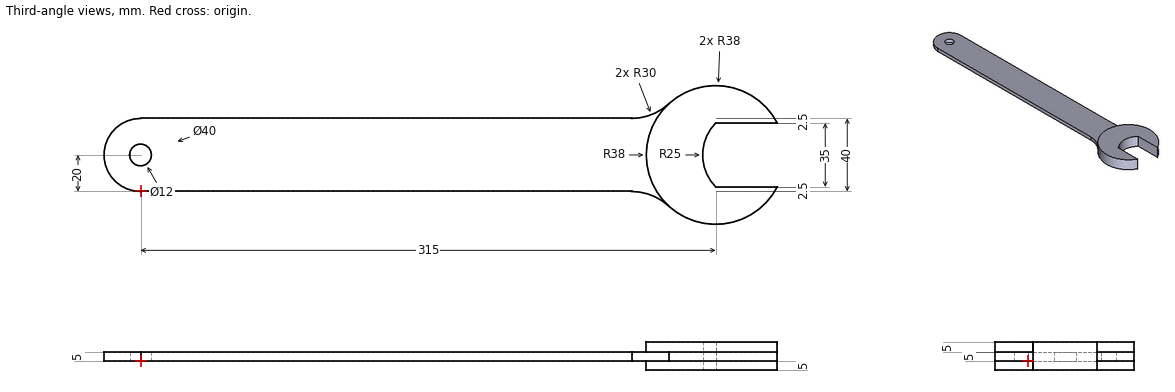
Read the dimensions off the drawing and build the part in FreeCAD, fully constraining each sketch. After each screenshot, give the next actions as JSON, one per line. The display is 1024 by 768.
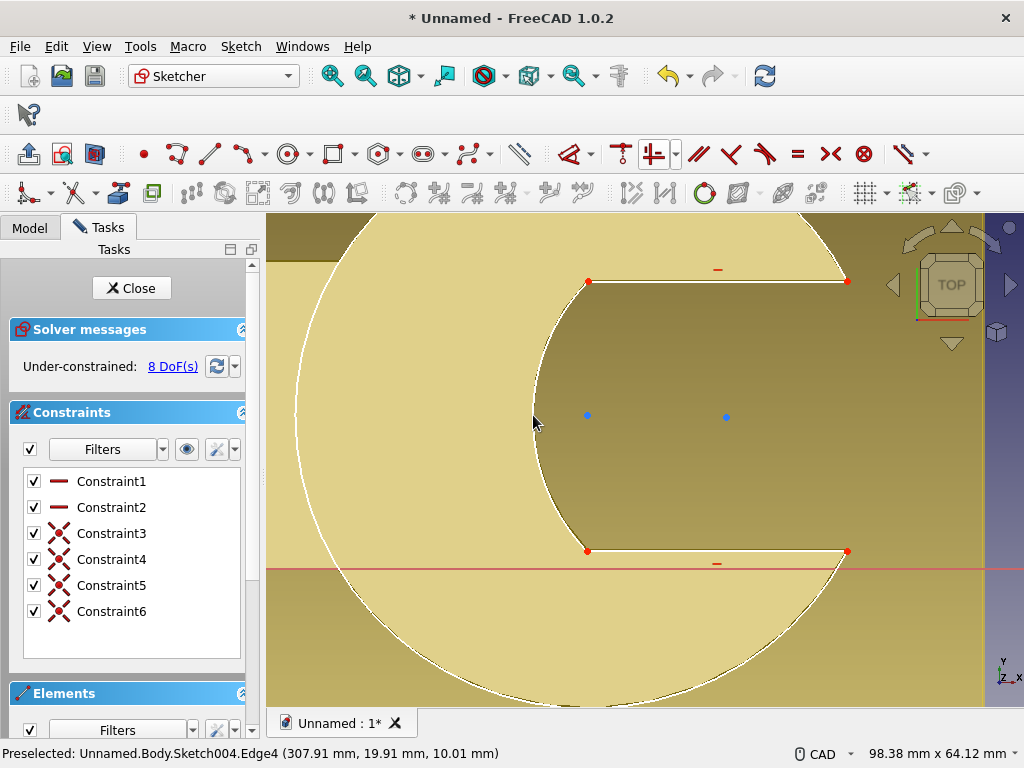
{"action": "left_click", "coordinate": [568, 154]}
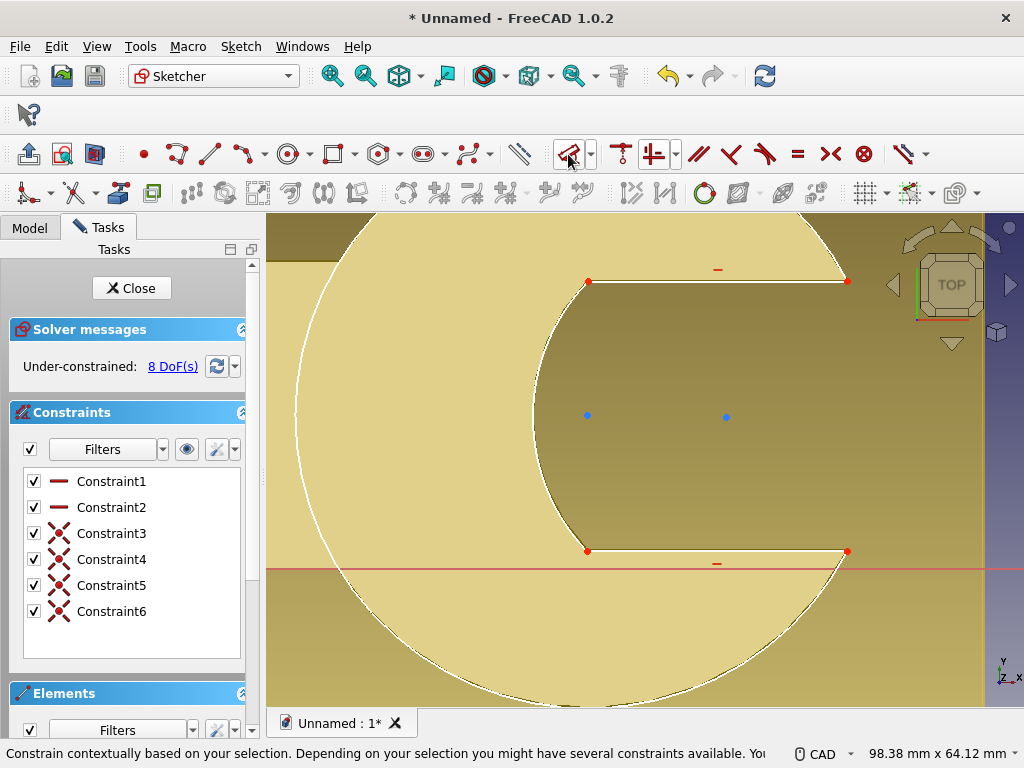
{"action": "left_click", "coordinate": [446, 671]}
{"action": "left_click", "coordinate": [314, 589]}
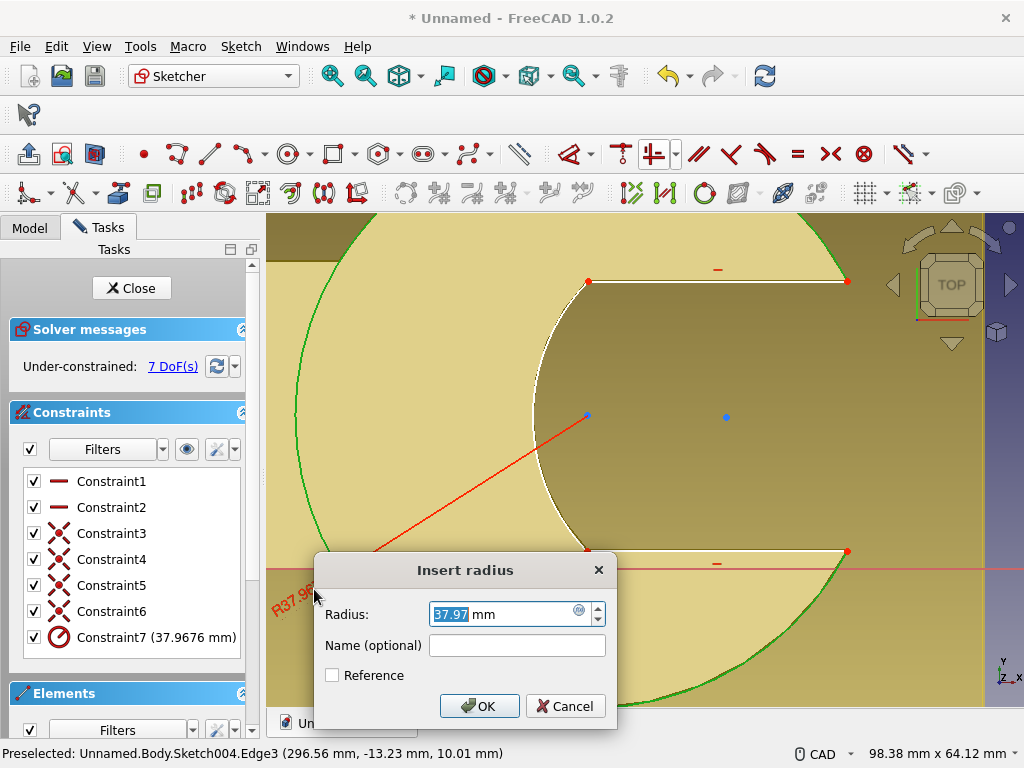
{"action": "type", "text": "38"}
{"action": "key", "text": "Return"}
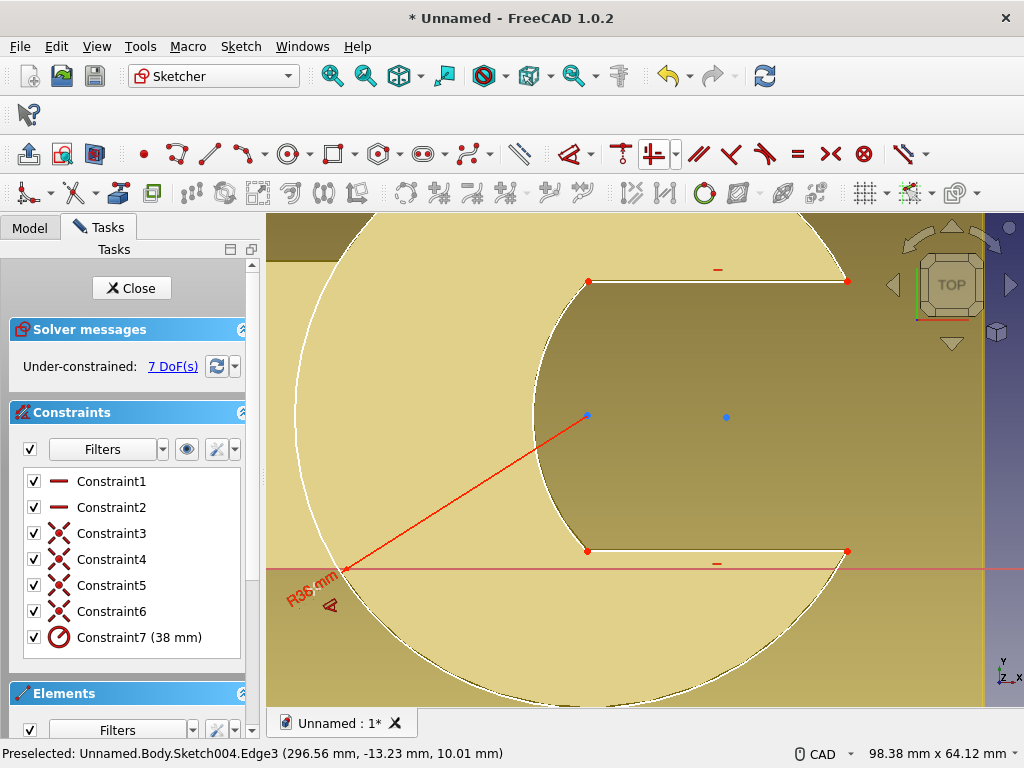
{"action": "left_click", "coordinate": [542, 358]}
{"action": "left_click", "coordinate": [512, 348]}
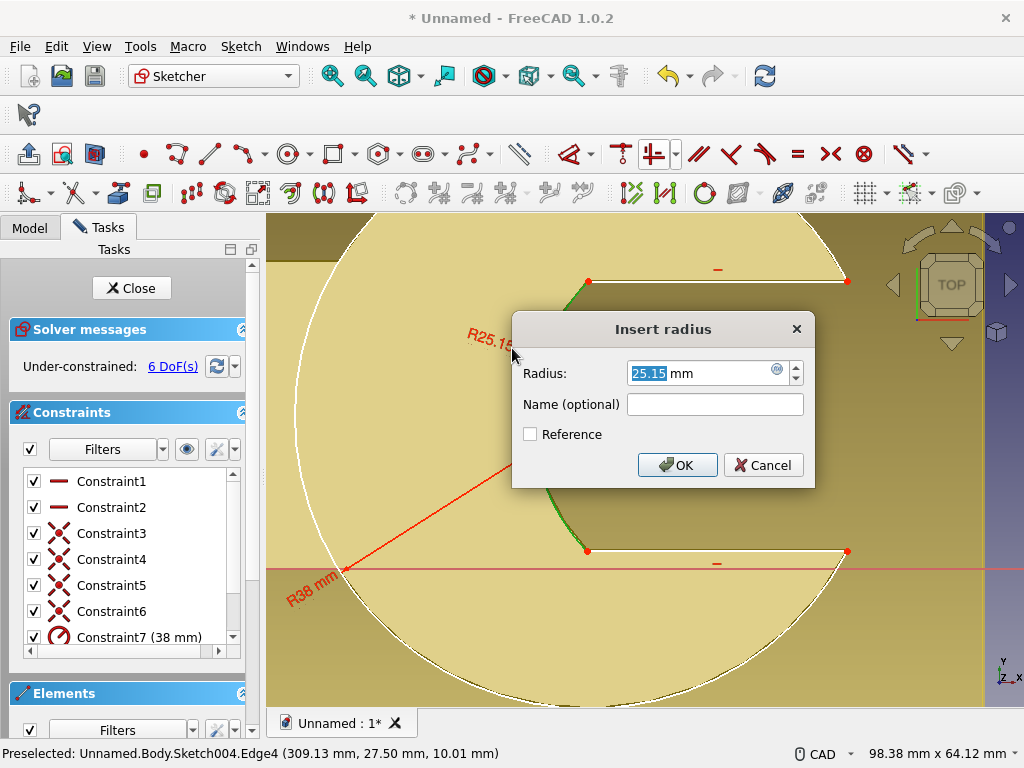
{"action": "type", "text": "25"}
{"action": "key", "text": "Return"}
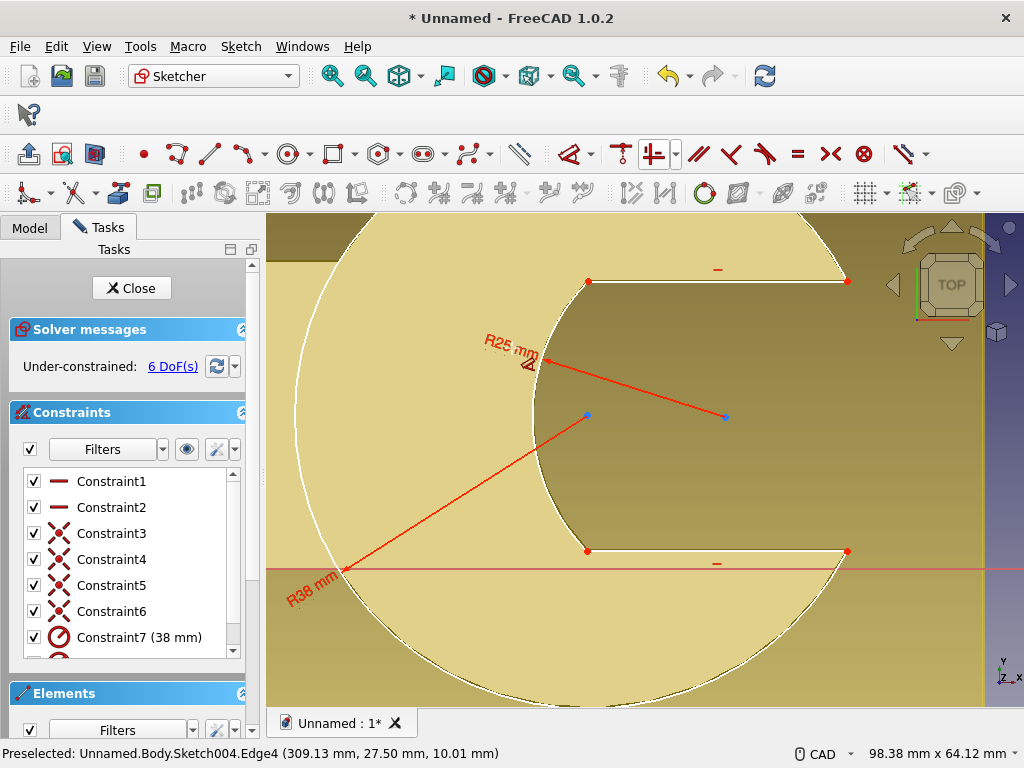
{"action": "left_click", "coordinate": [588, 416]}
{"action": "left_click", "coordinate": [622, 493]}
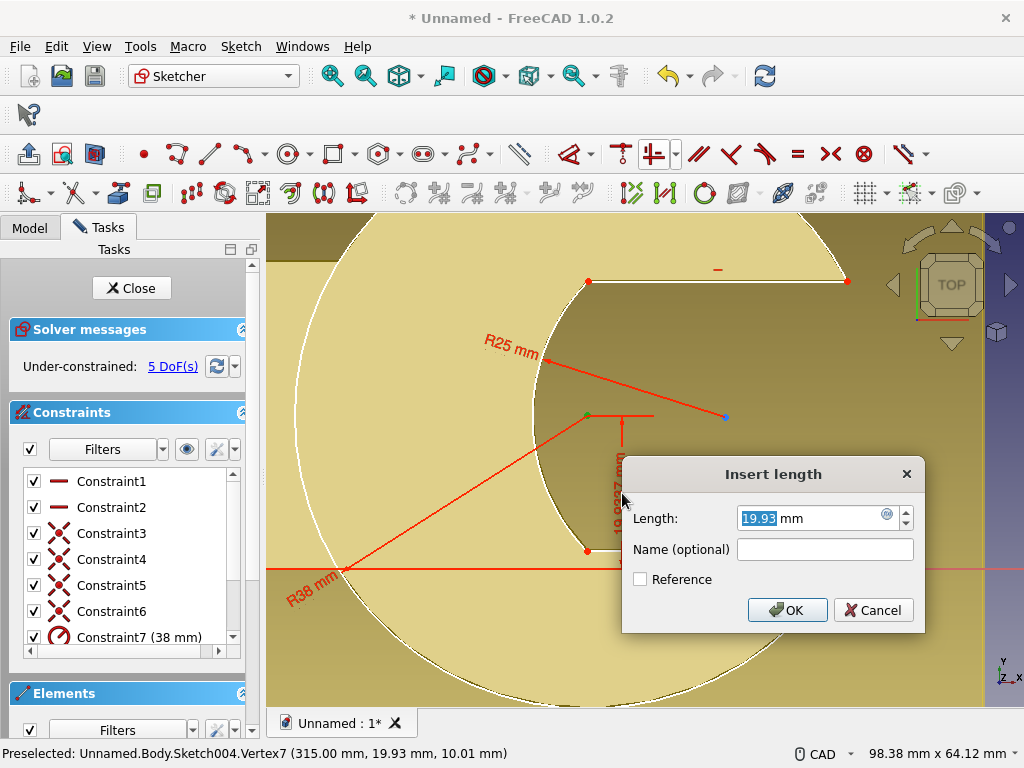
{"action": "type", "text": "20"}
{"action": "key", "text": "Return"}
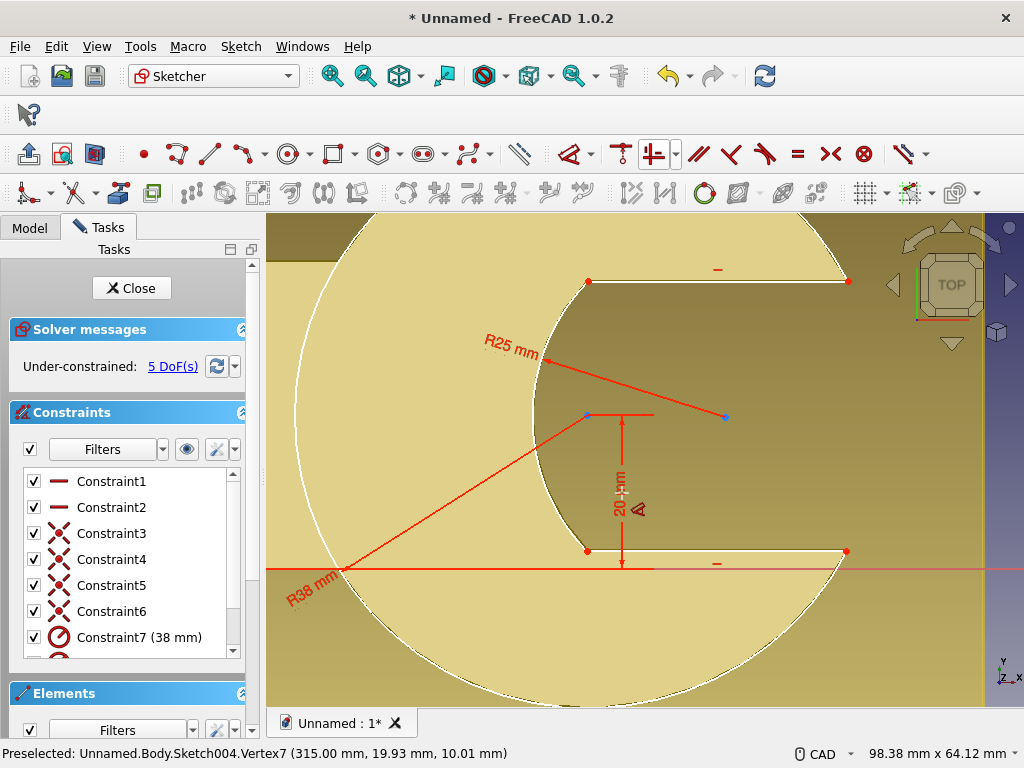
{"action": "left_click", "coordinate": [725, 417]}
{"action": "left_click", "coordinate": [759, 493]}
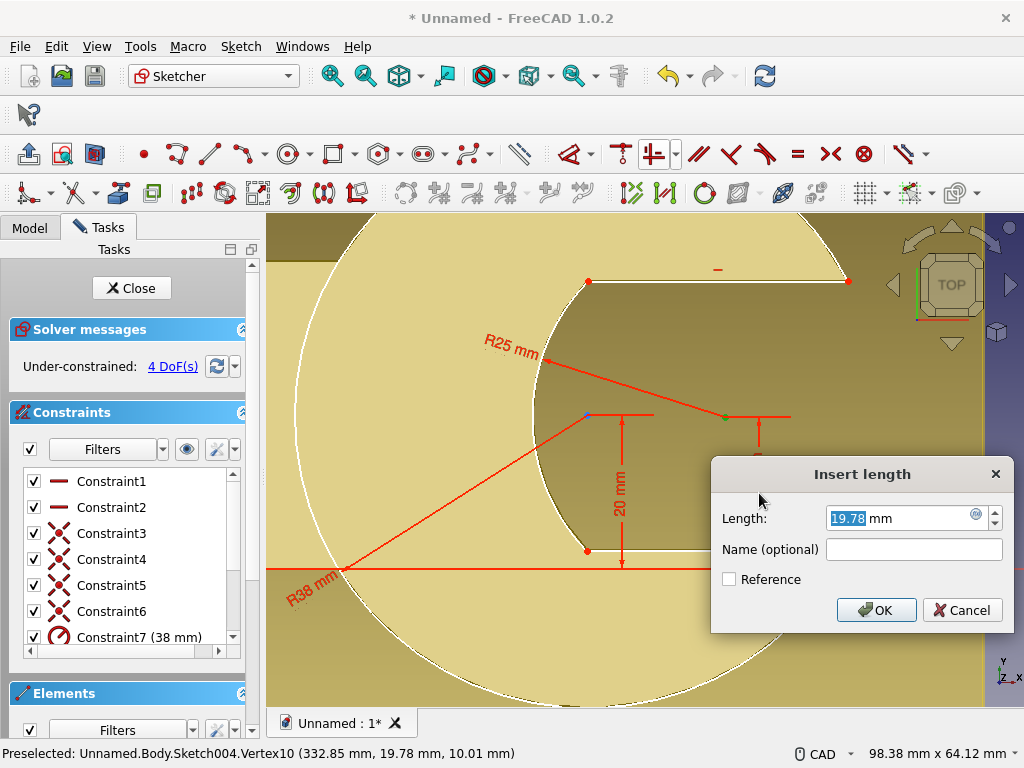
{"action": "type", "text": "20"}
{"action": "key", "text": "Return"}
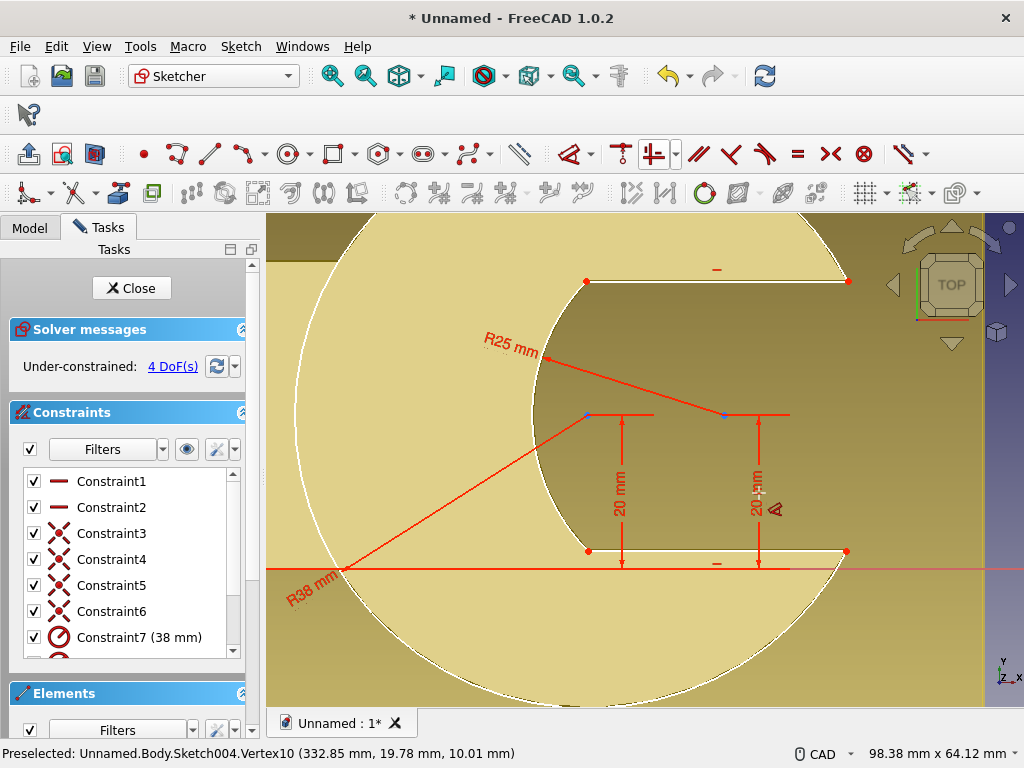
{"action": "left_click", "coordinate": [586, 282]}
{"action": "left_click", "coordinate": [440, 603]}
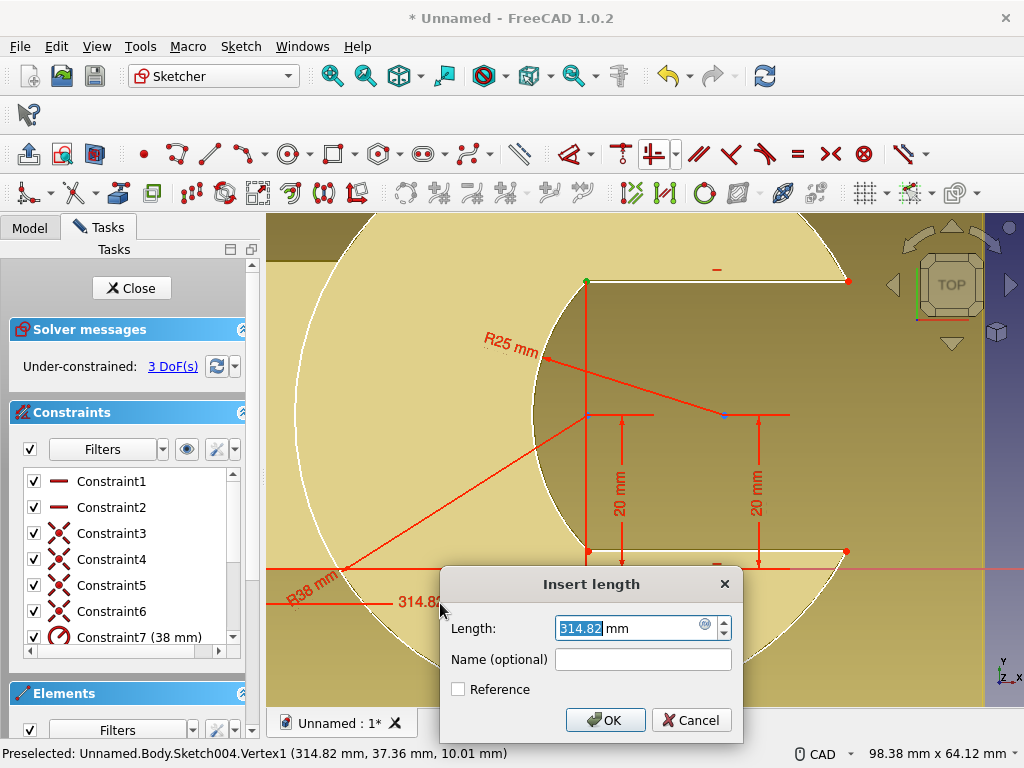
{"action": "type", "text": "315"}
{"action": "key", "text": "Return"}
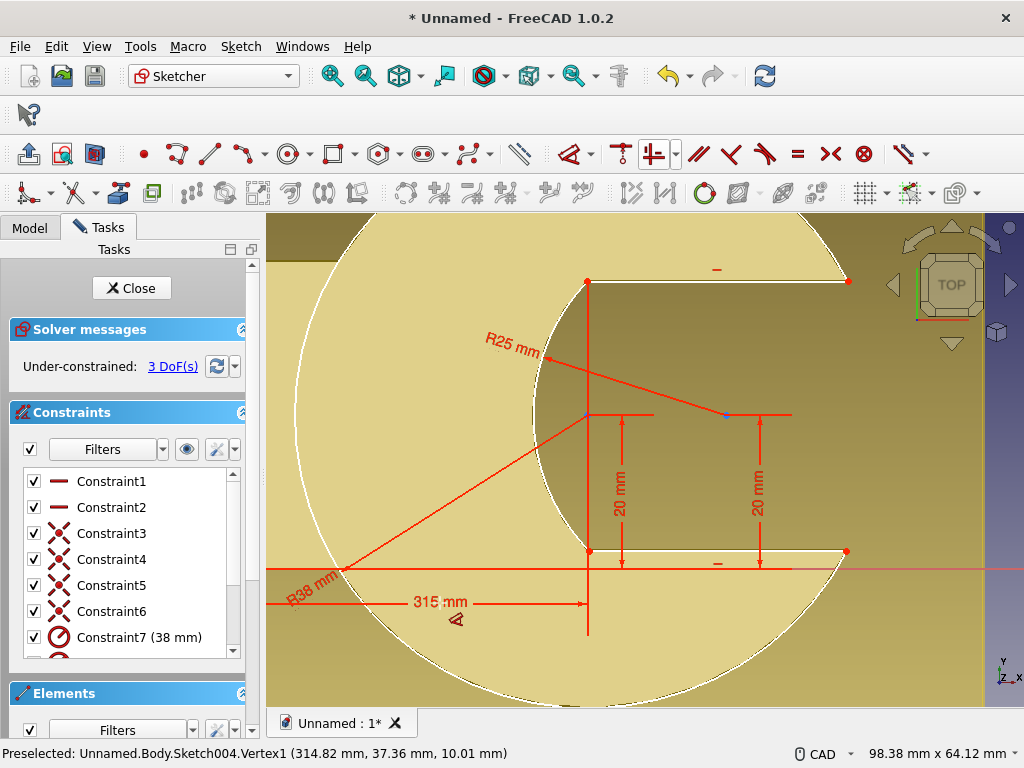
{"action": "scroll", "coordinate": [847, 551], "scroll_direction": "up", "scroll_amount": 4}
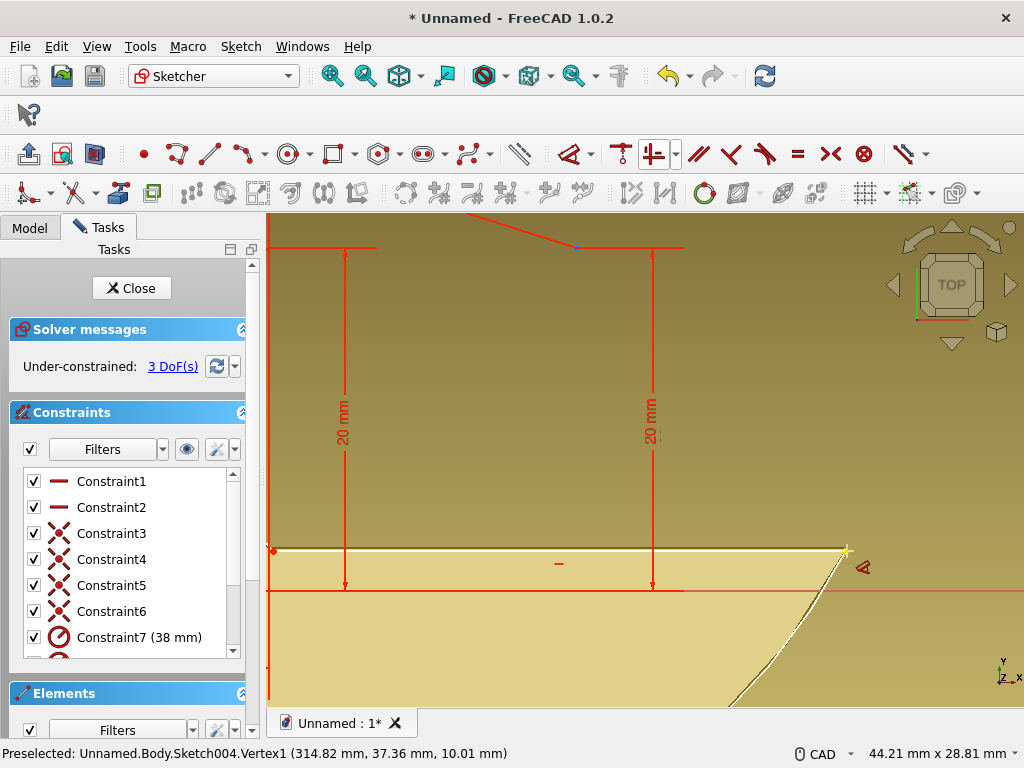
{"action": "left_click", "coordinate": [846, 551]}